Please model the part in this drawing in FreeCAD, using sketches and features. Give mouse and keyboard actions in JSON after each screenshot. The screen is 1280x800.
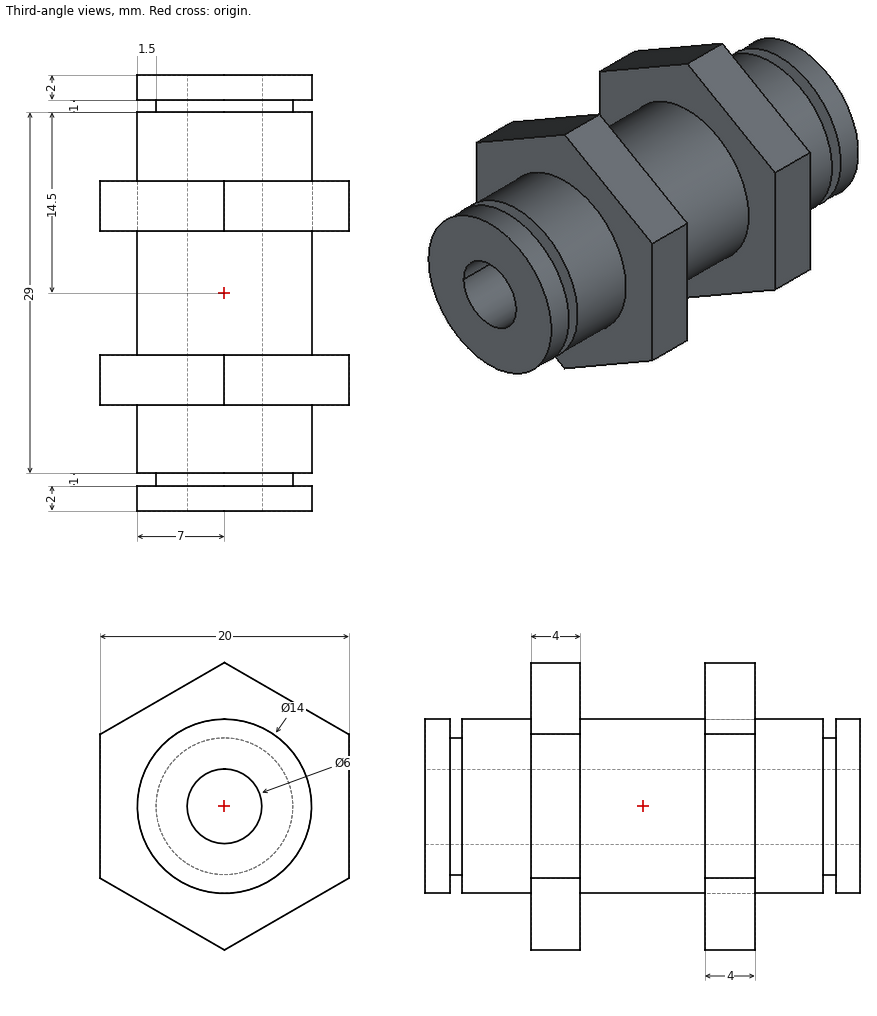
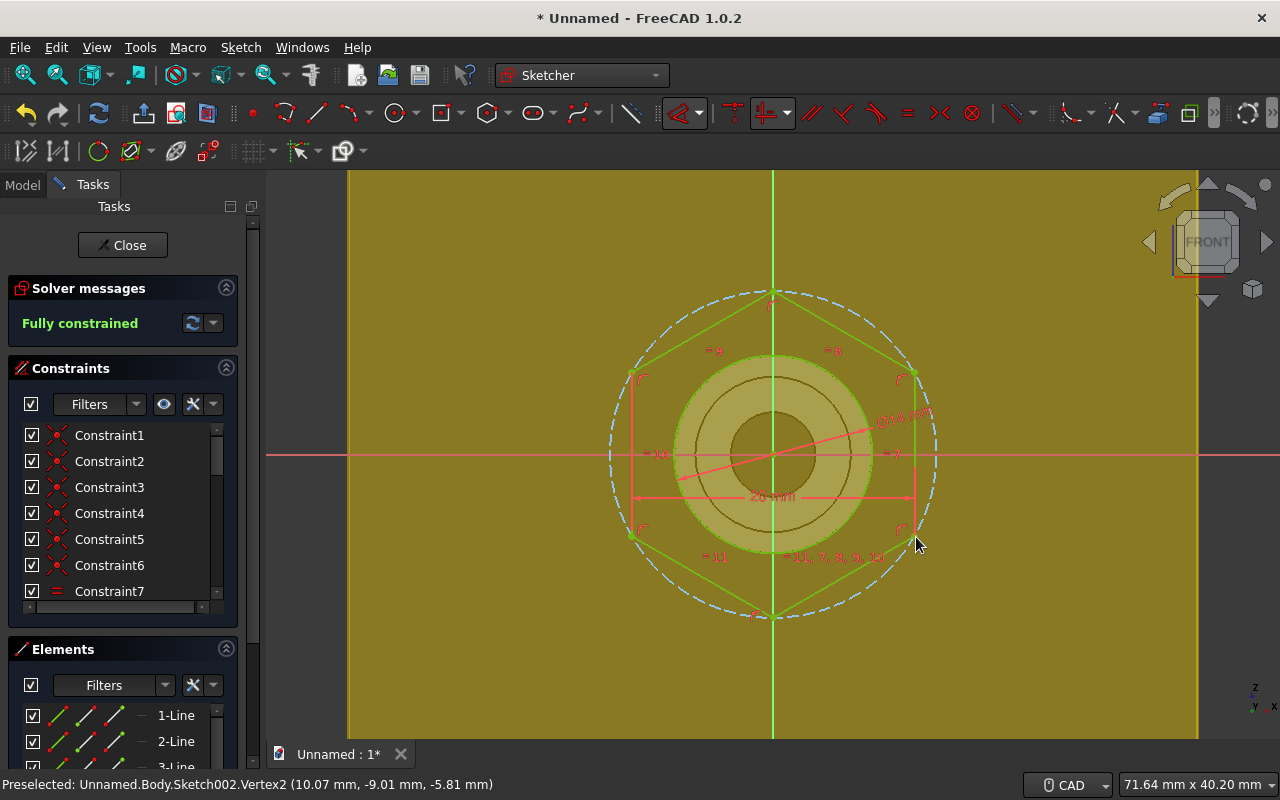
{"action": "left_click", "coordinate": [123, 245]}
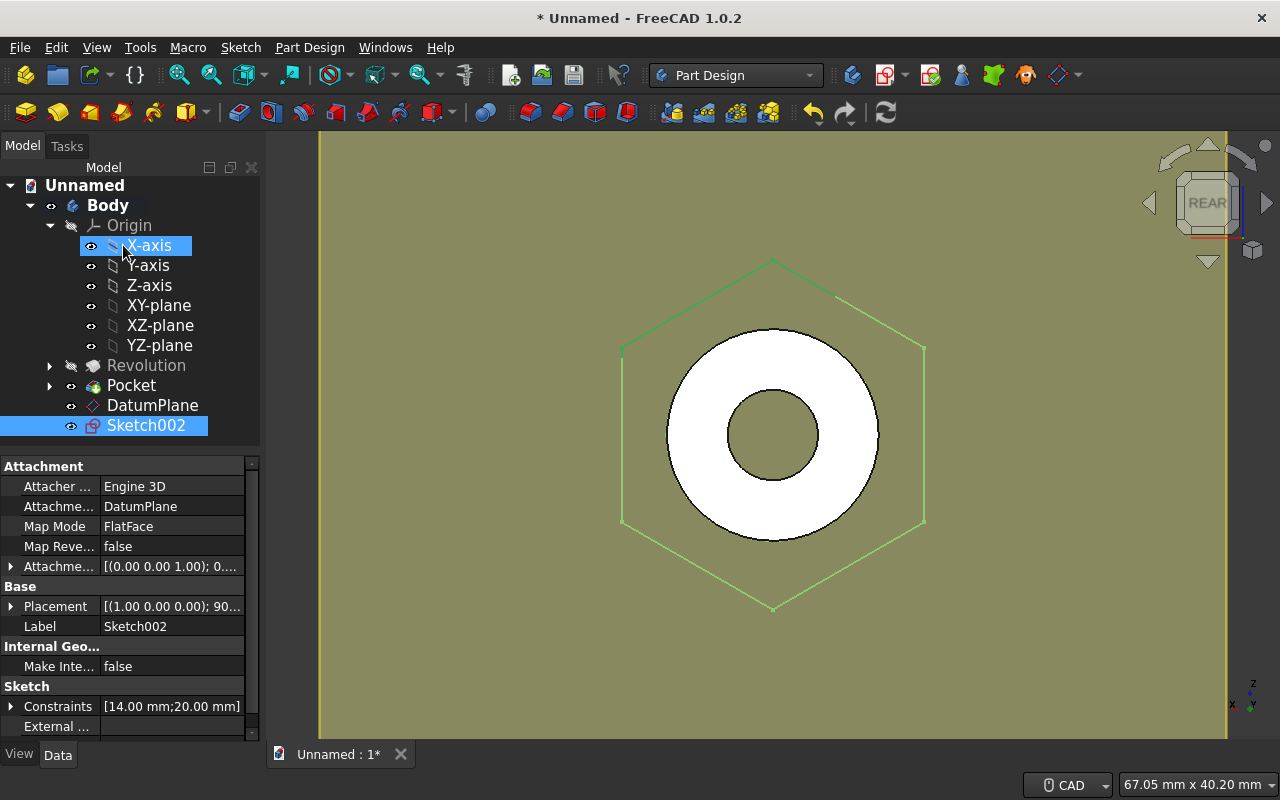
{"action": "left_click", "coordinate": [26, 112]}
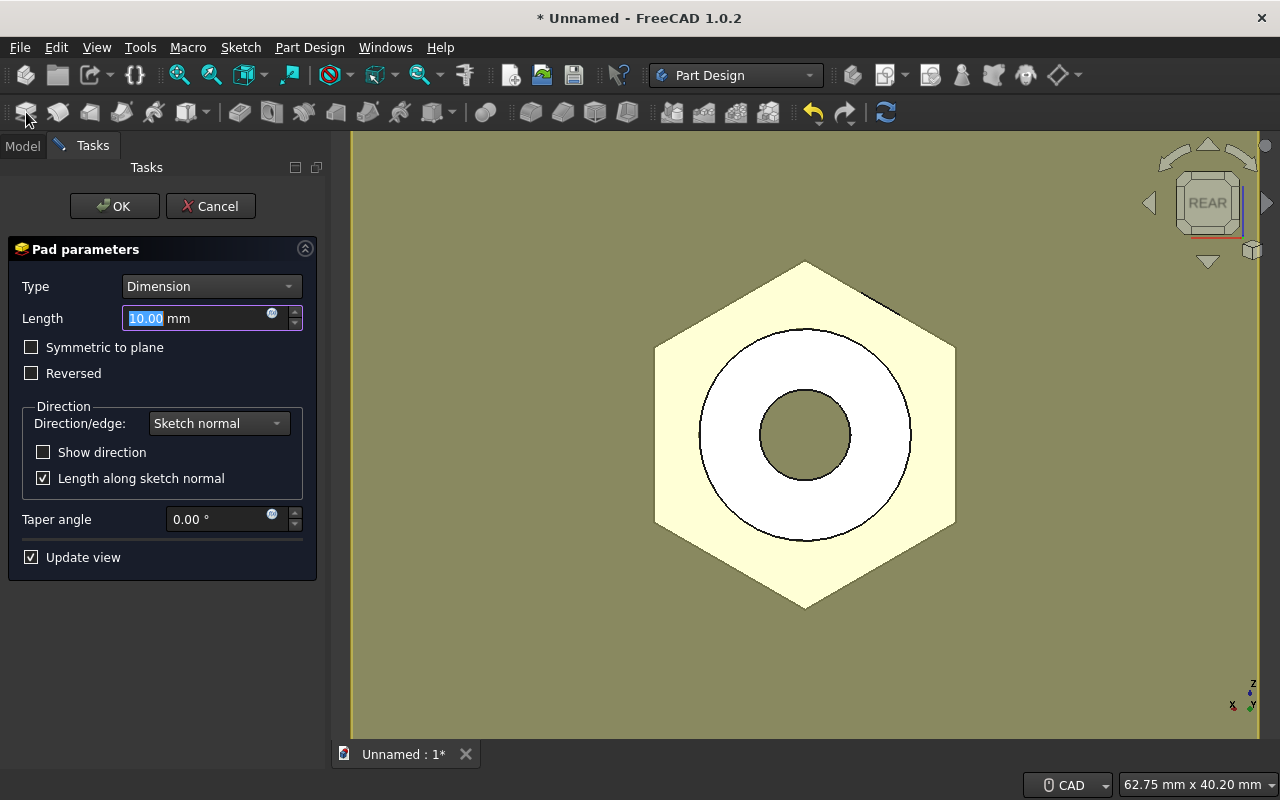
{"action": "type", "text": "4"}
{"action": "key", "text": "Tab"}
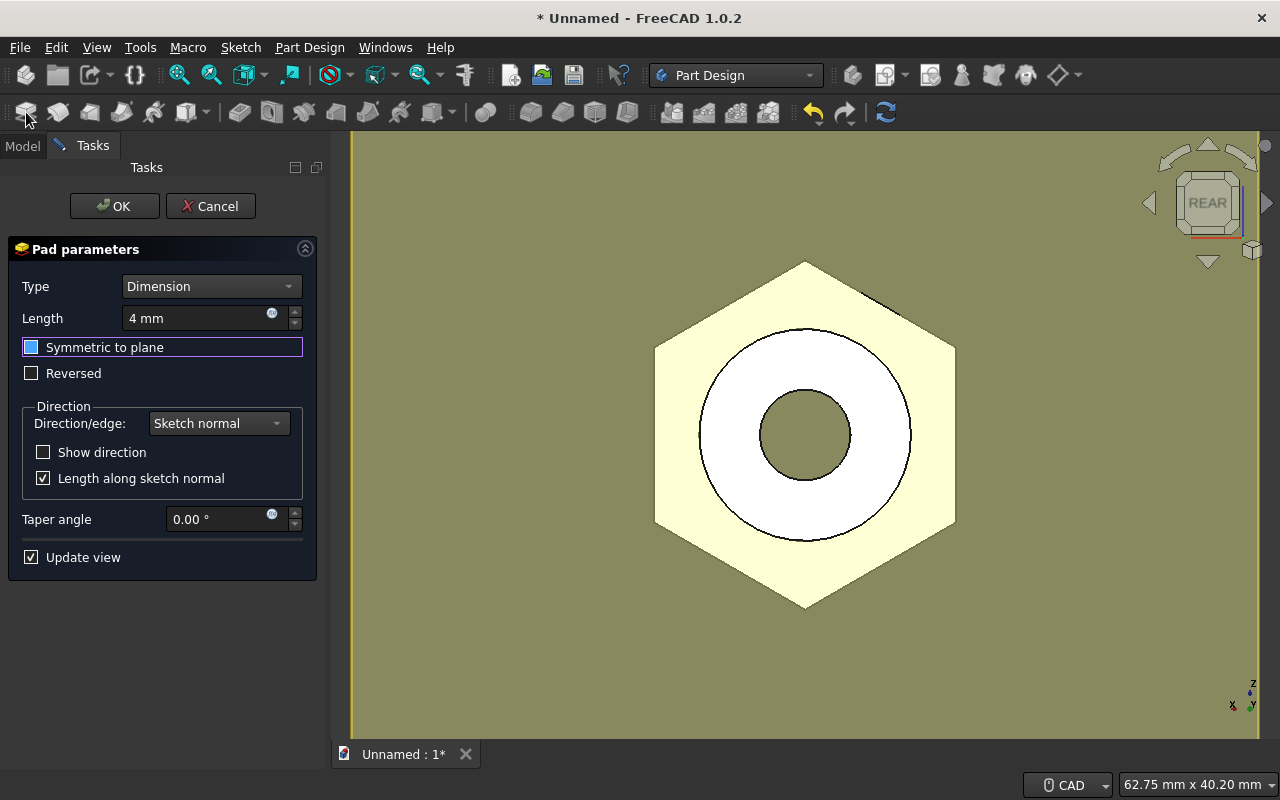
{"action": "left_click", "coordinate": [30, 373]}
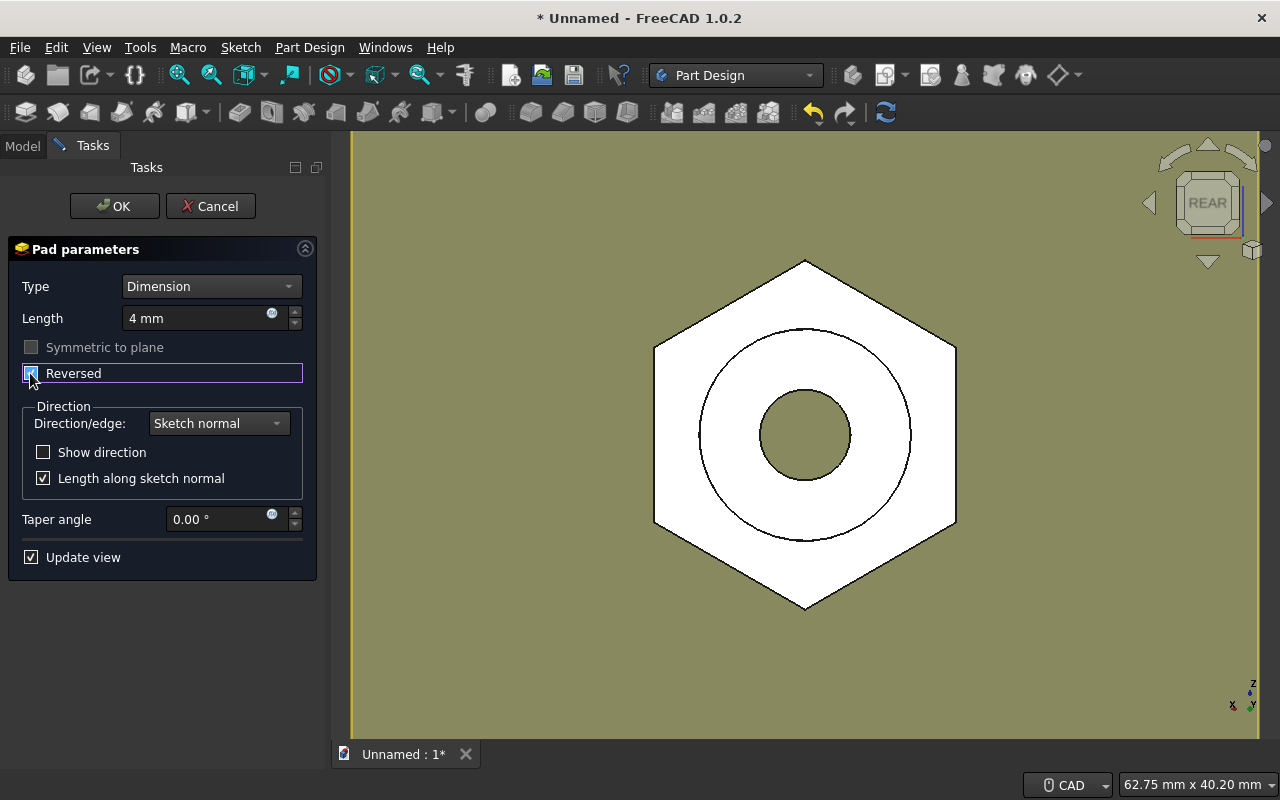
{"action": "left_click", "coordinate": [115, 206]}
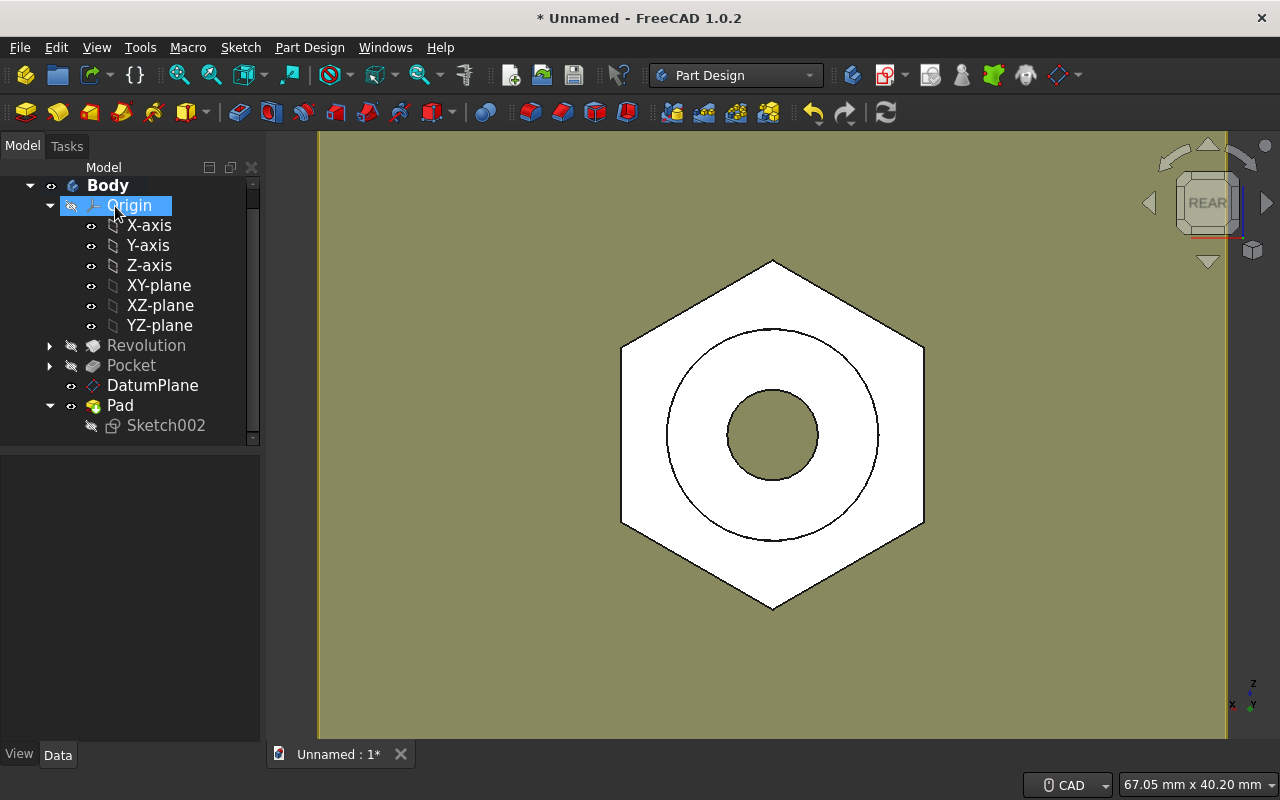
{"action": "left_click", "coordinate": [116, 386]}
{"action": "key", "text": "space"}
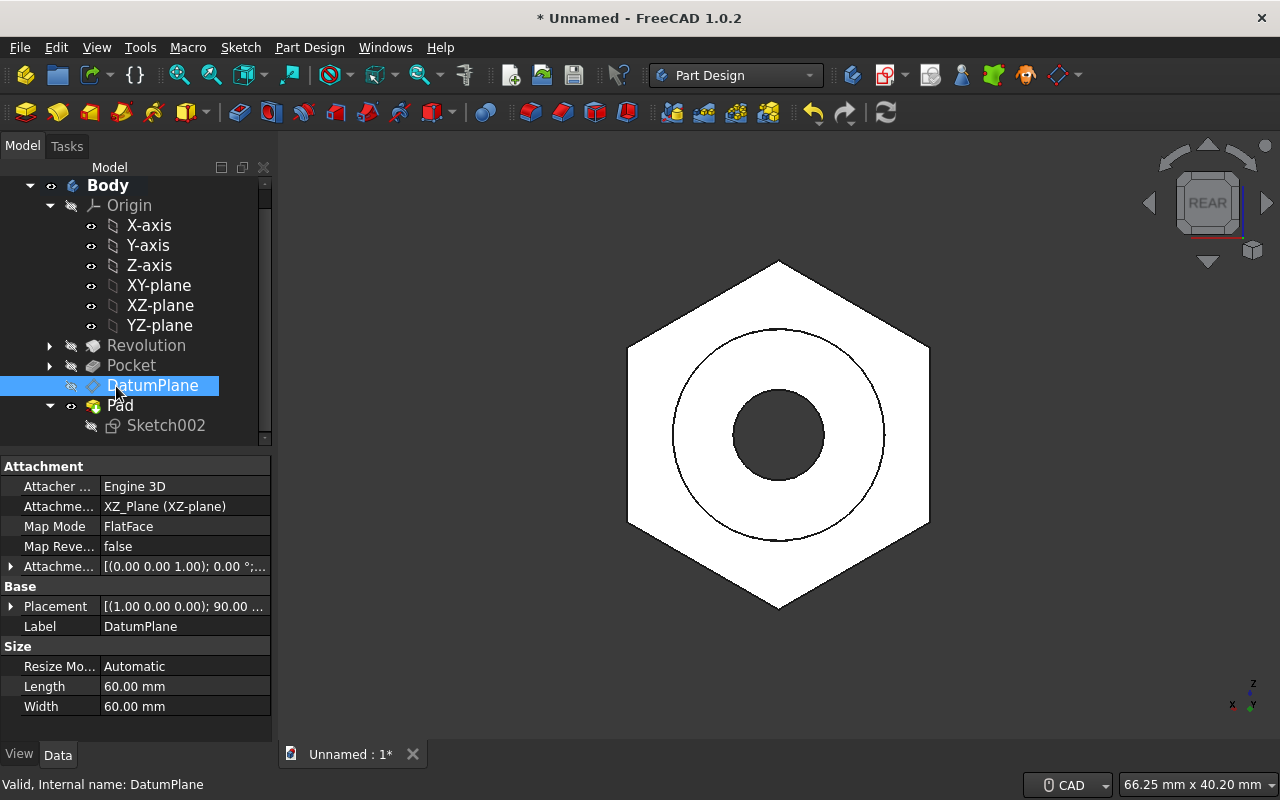
{"action": "left_click", "coordinate": [318, 699]}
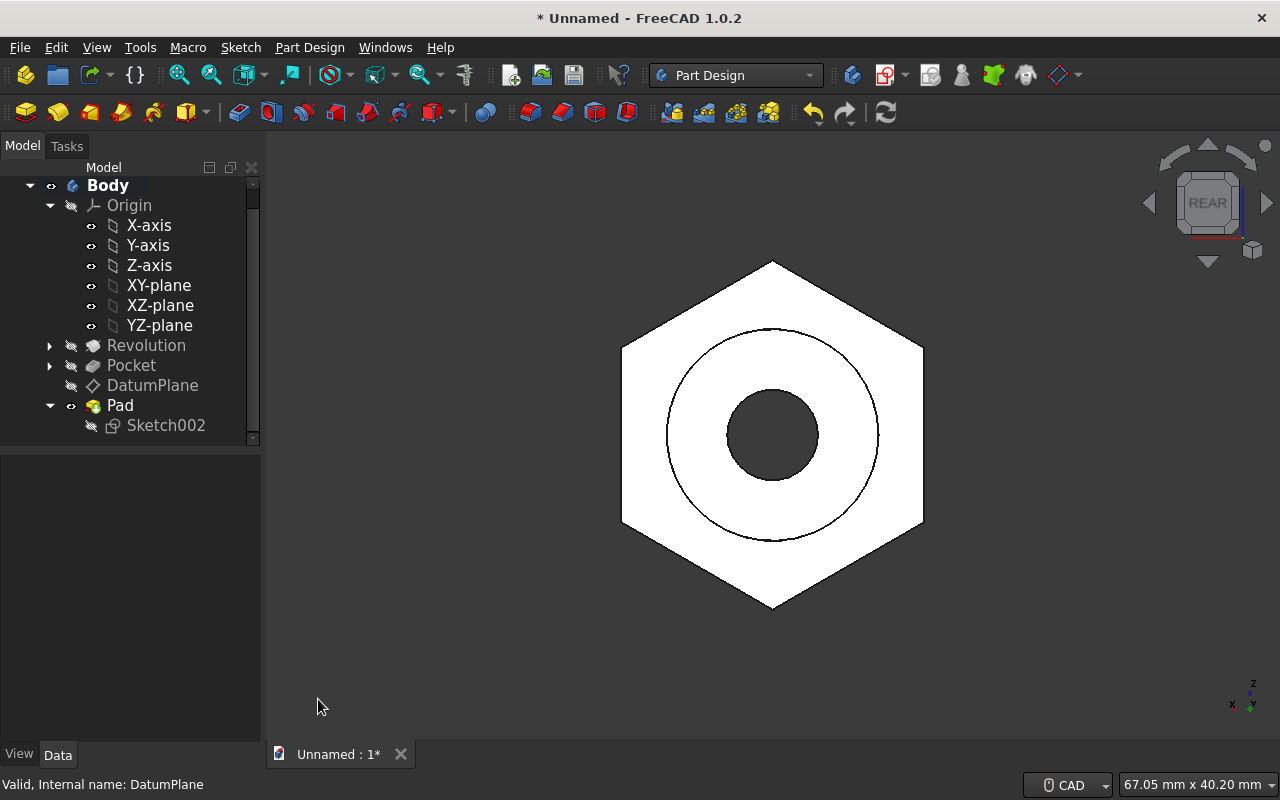
{"action": "left_click", "coordinate": [854, 76]}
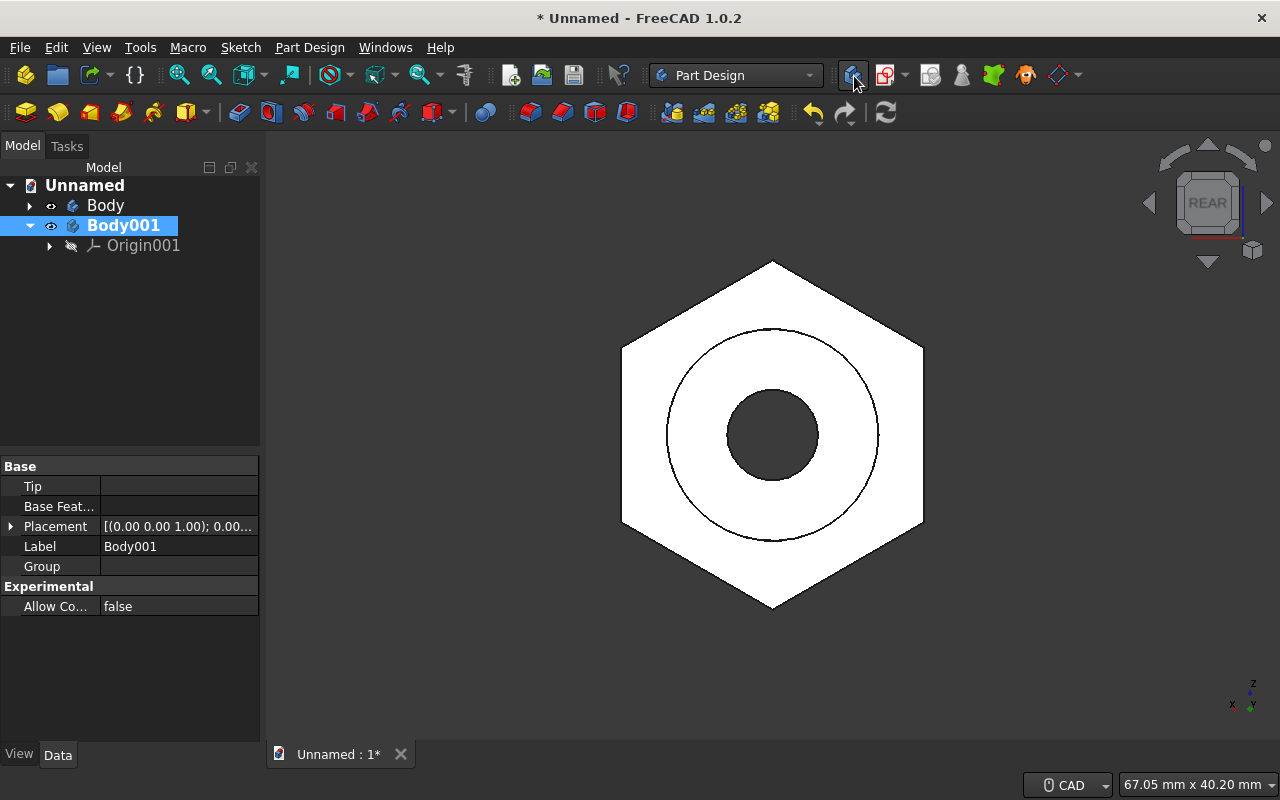
{"action": "left_click", "coordinate": [50, 246]}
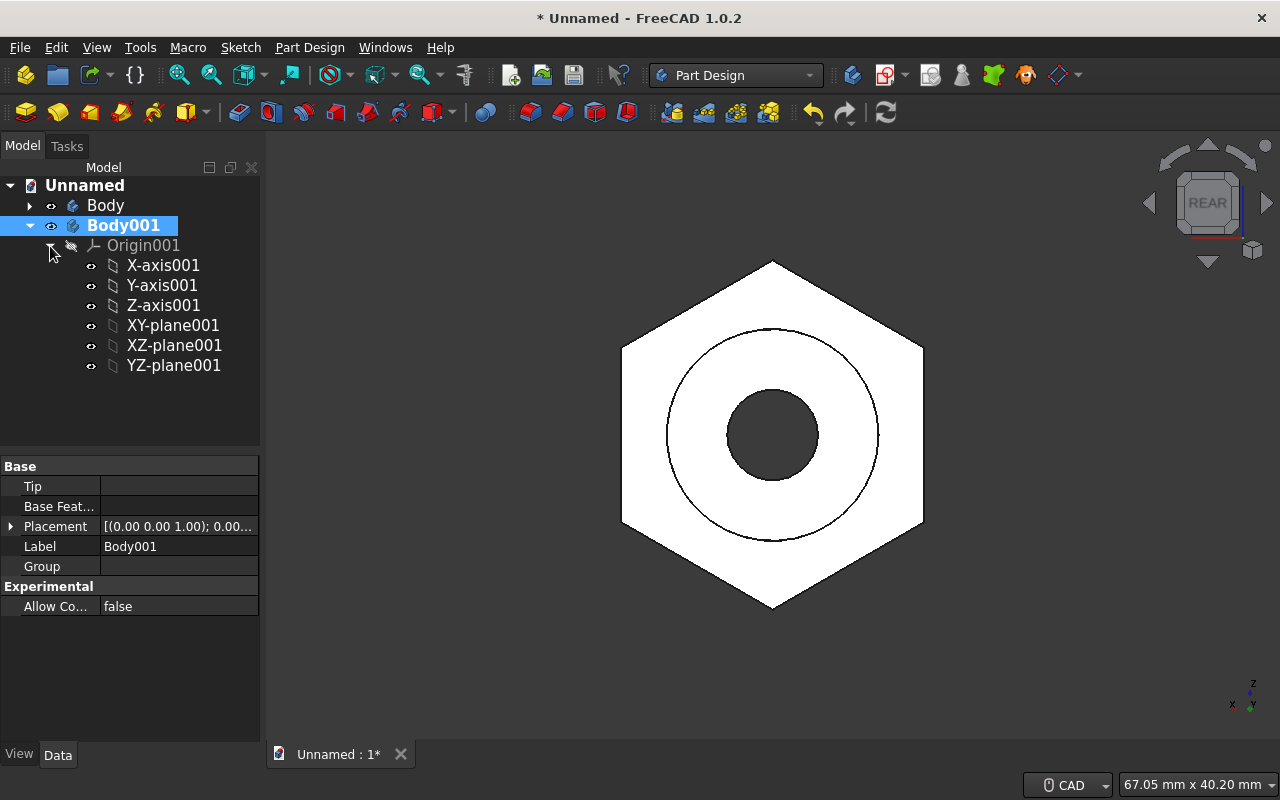
{"action": "left_click", "coordinate": [136, 346]}